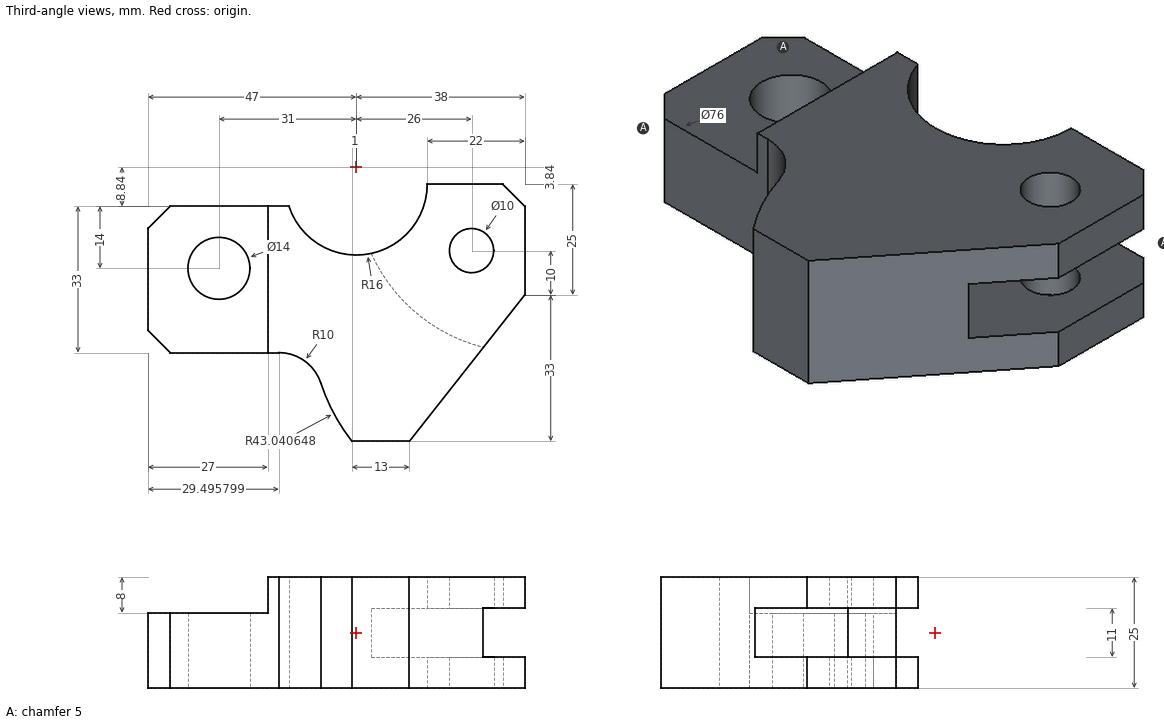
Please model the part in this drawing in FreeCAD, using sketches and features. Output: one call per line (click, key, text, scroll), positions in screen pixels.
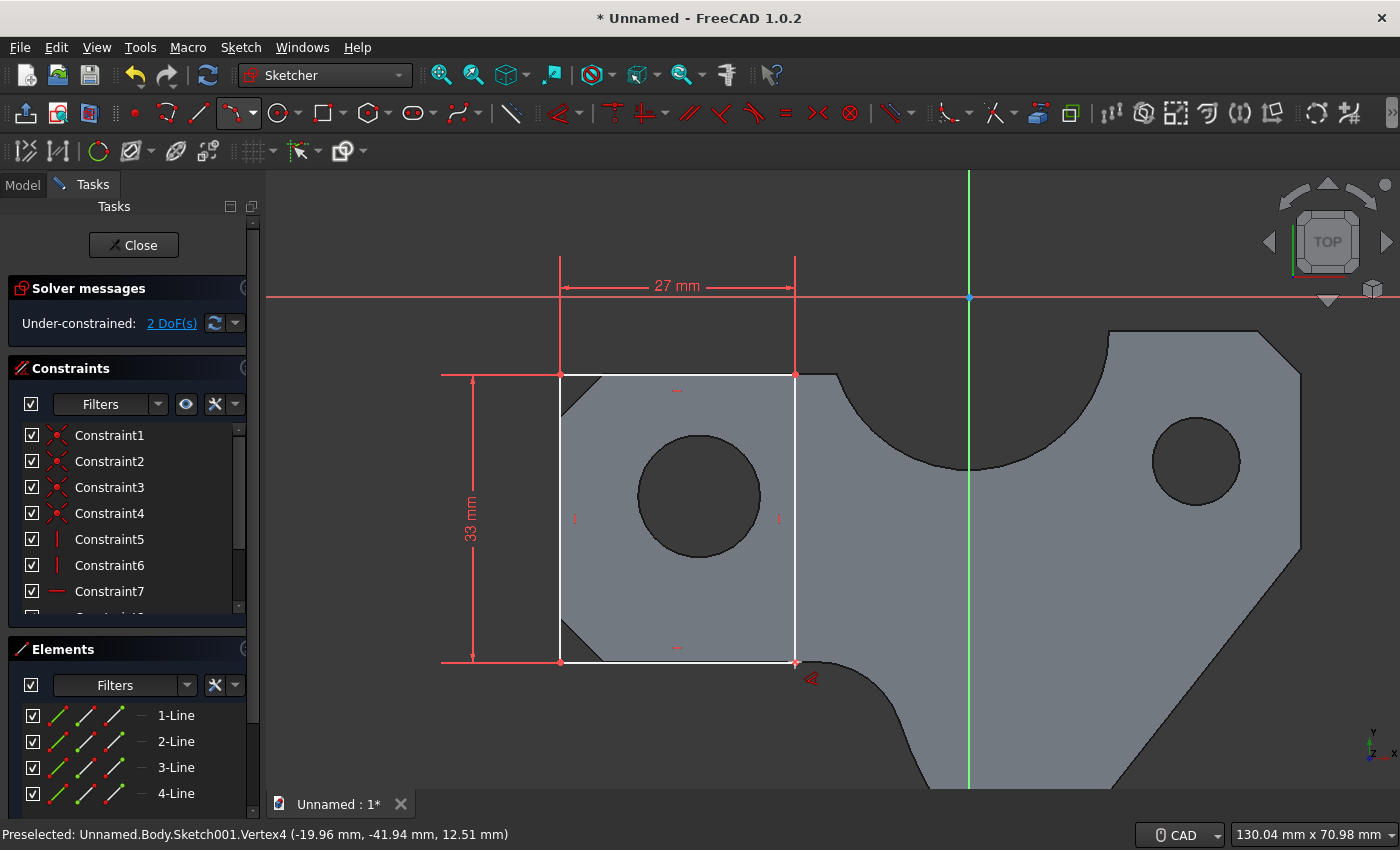
click(560, 375)
click(765, 263)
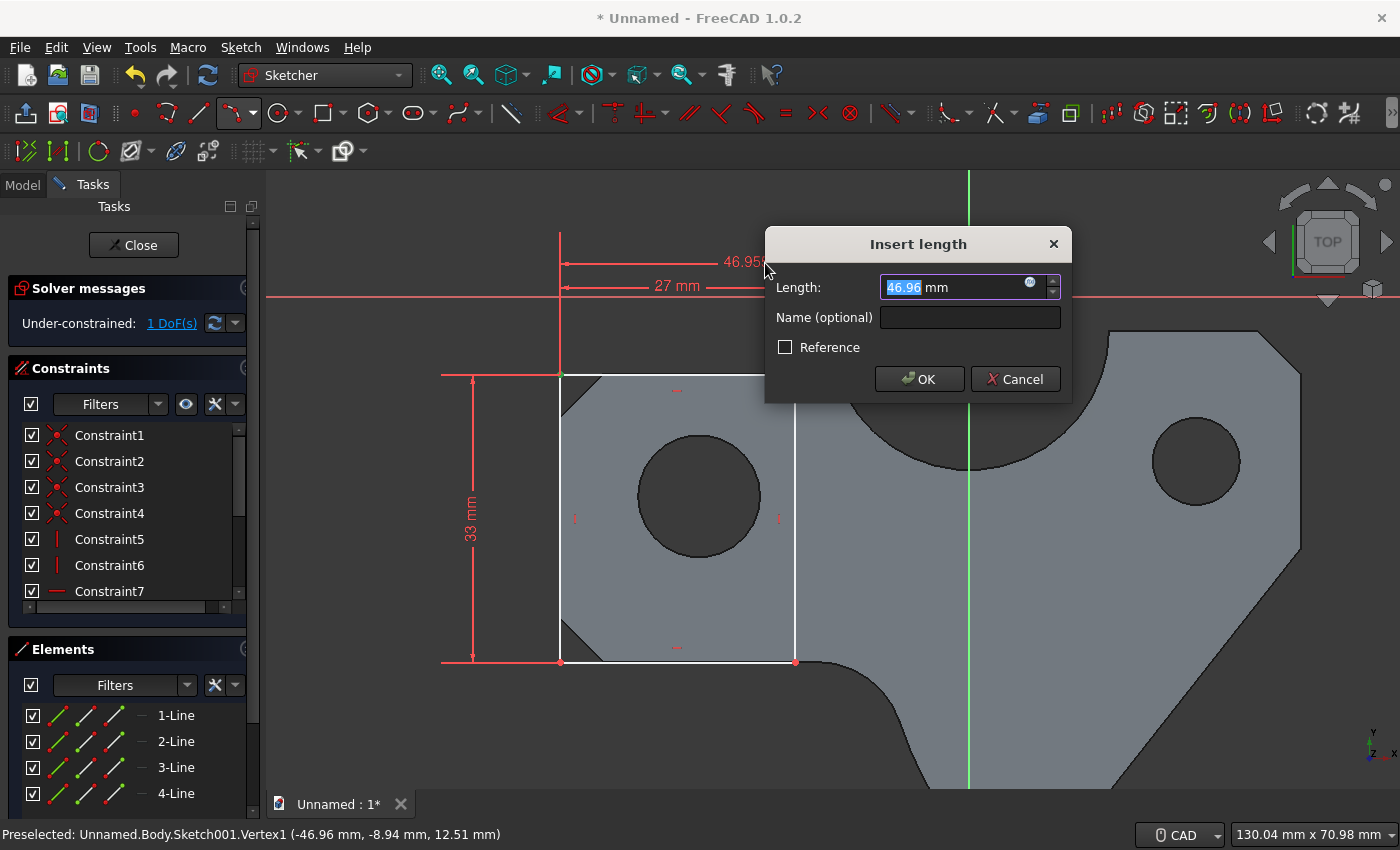
text(47)
key(Return)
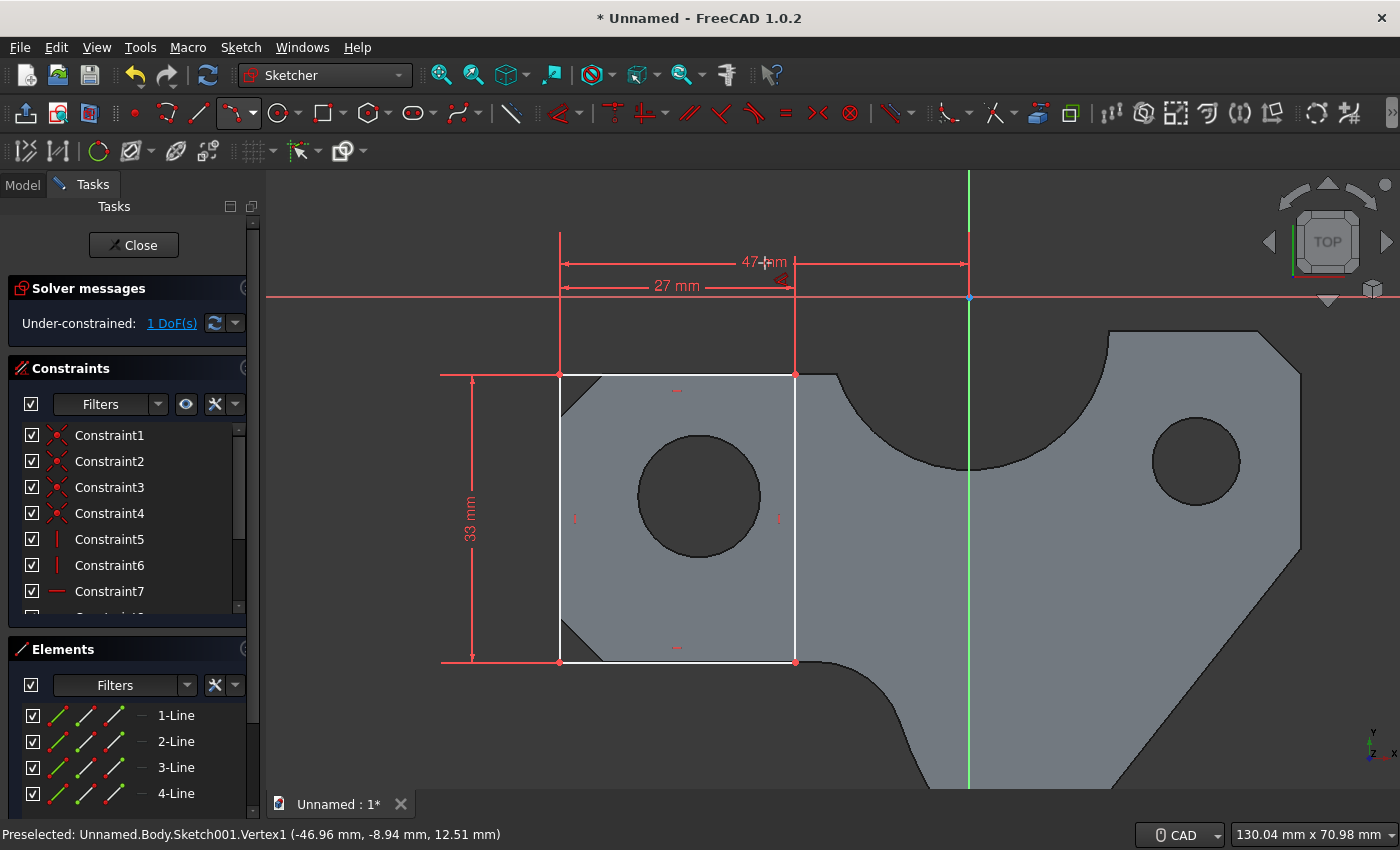
click(560, 375)
click(1003, 336)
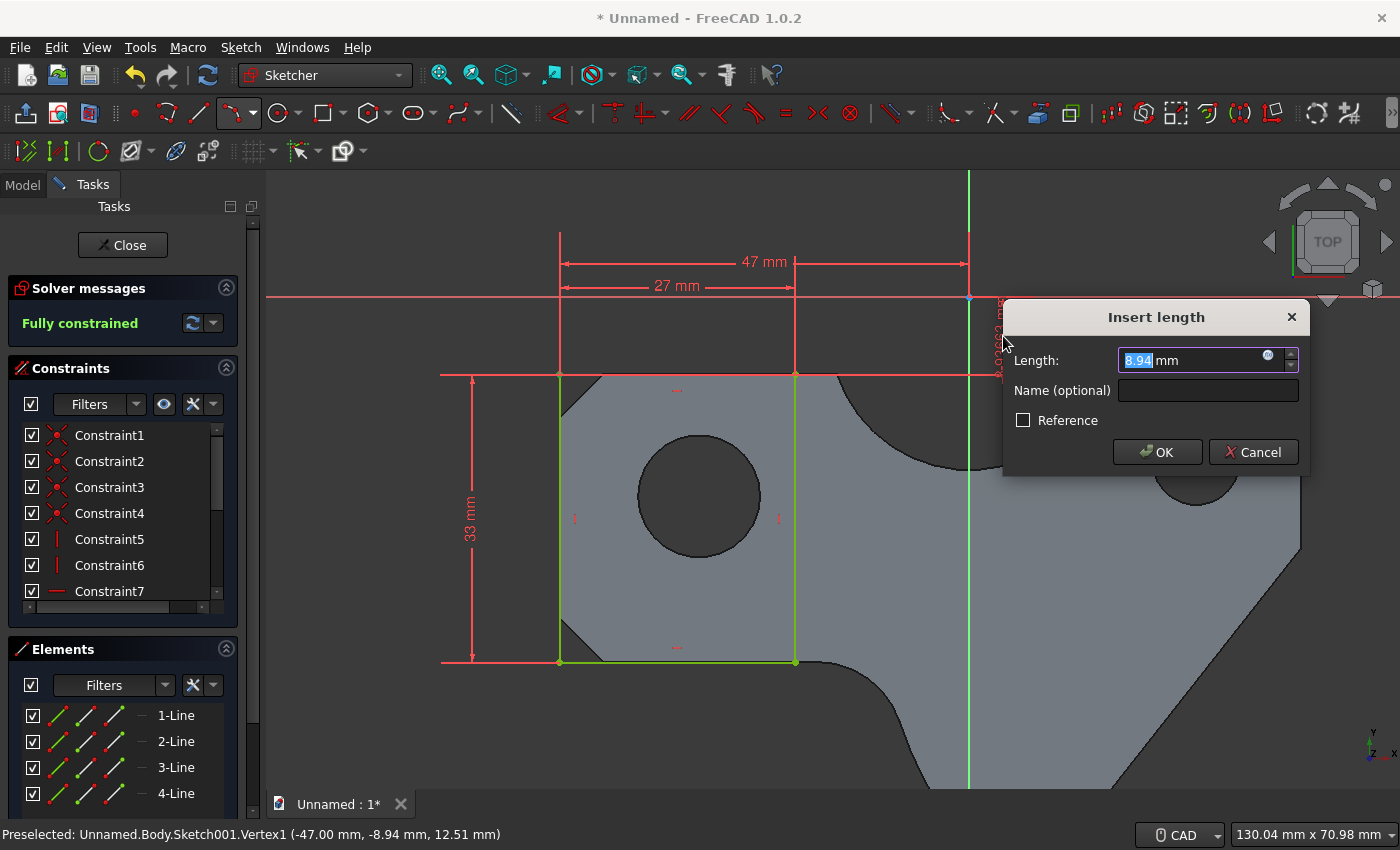
text(8.84)
key(Return)
key(Escape)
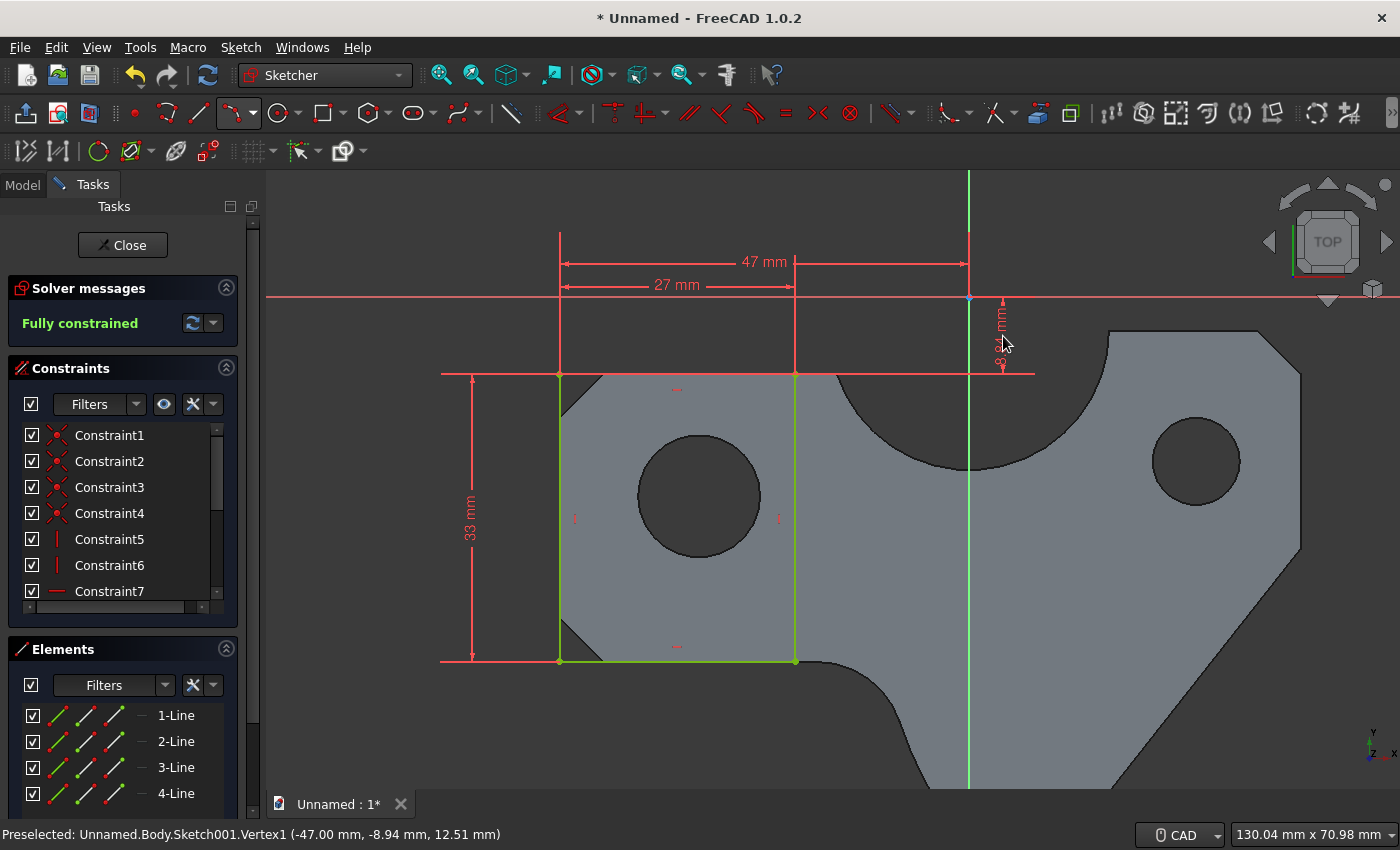
click(123, 245)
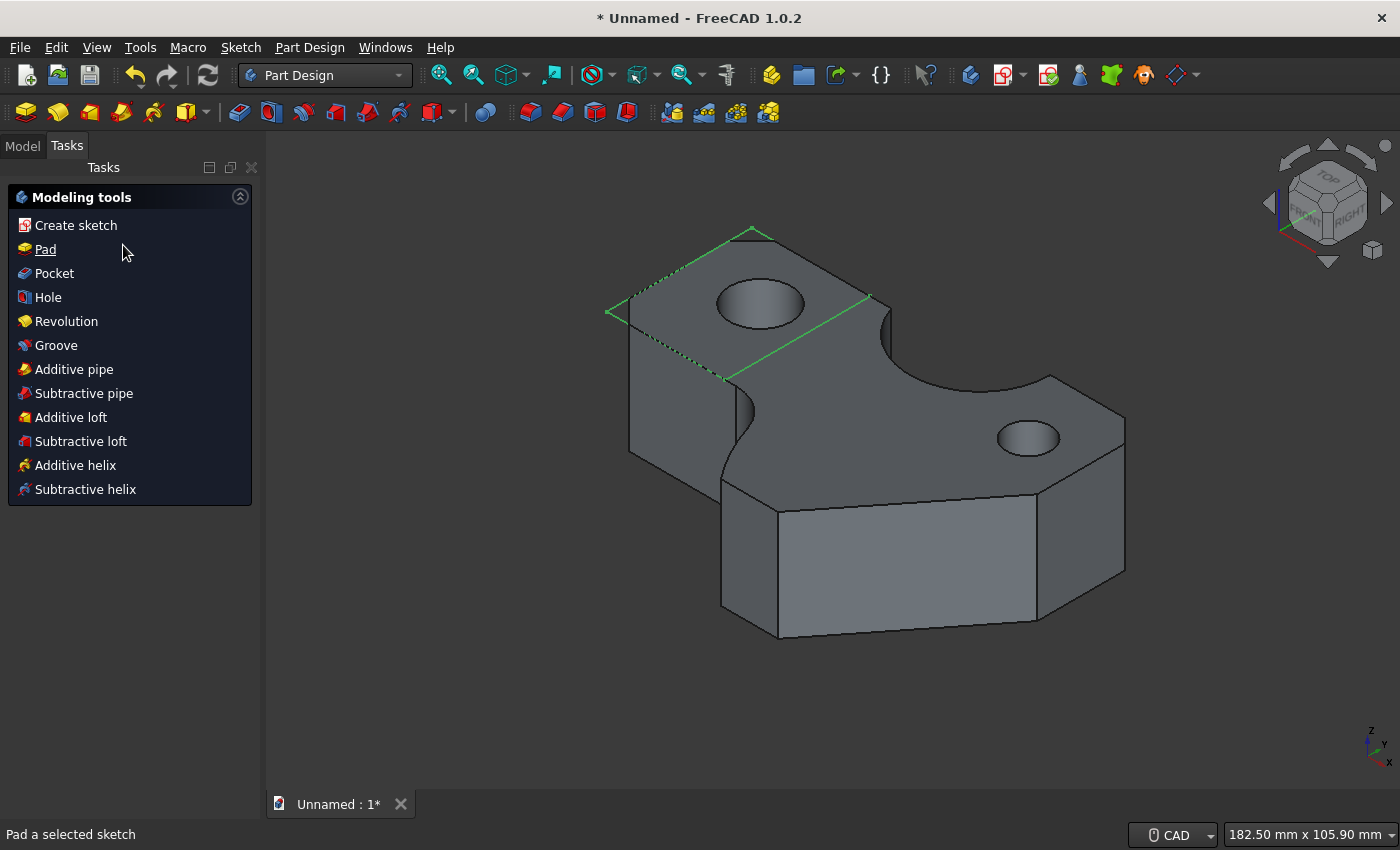
click(240, 112)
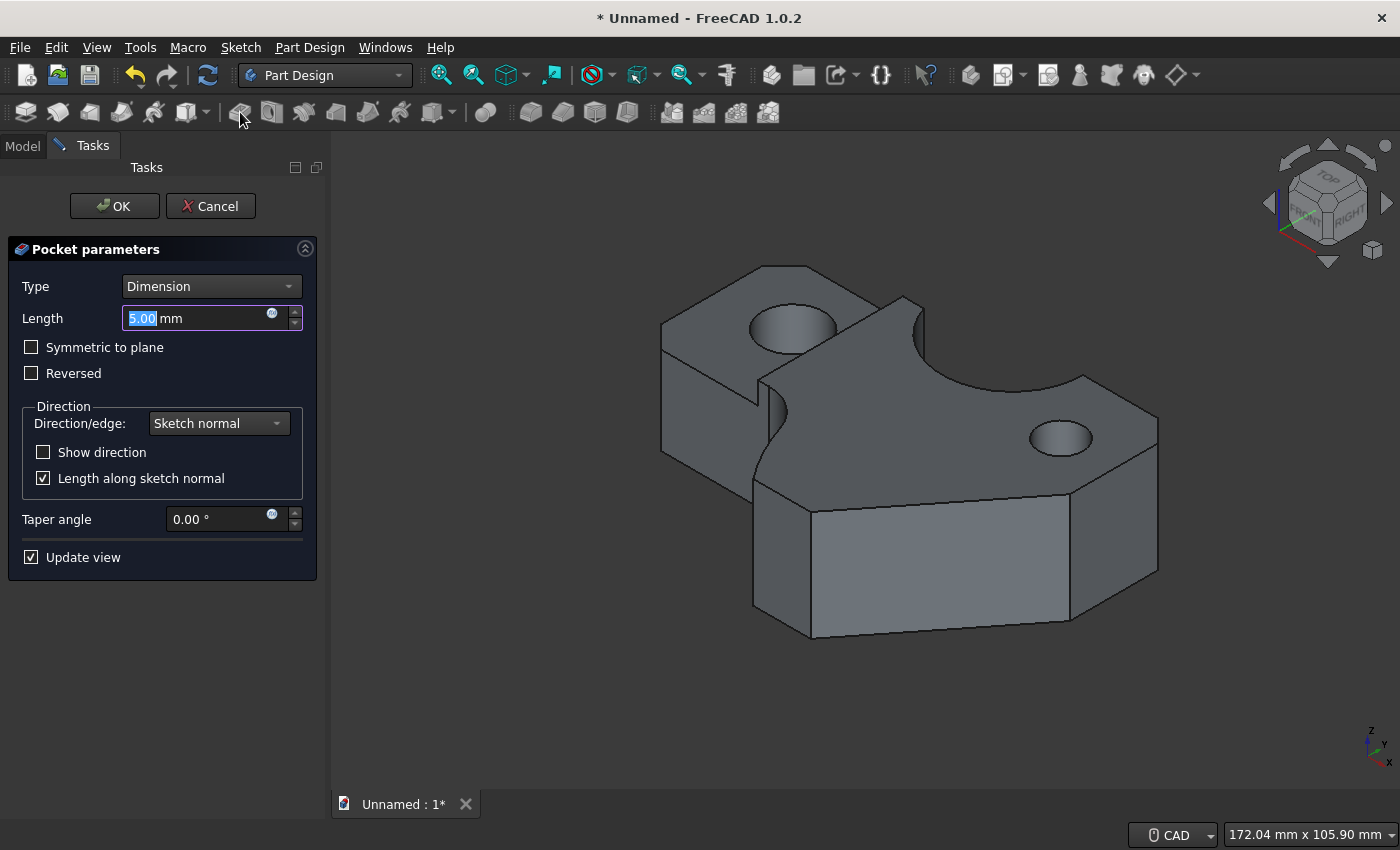
text(8)
key(Tab)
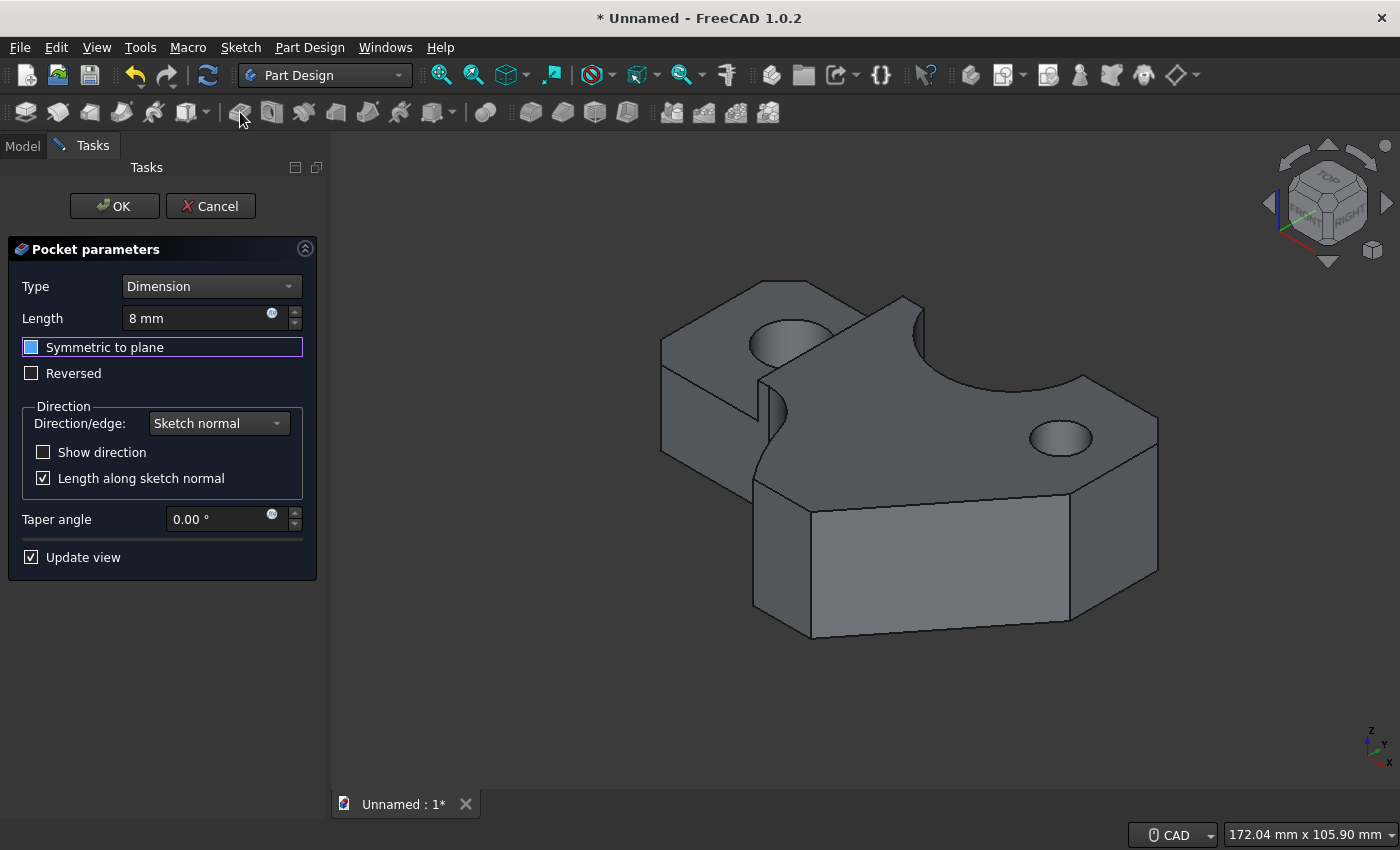
click(115, 206)